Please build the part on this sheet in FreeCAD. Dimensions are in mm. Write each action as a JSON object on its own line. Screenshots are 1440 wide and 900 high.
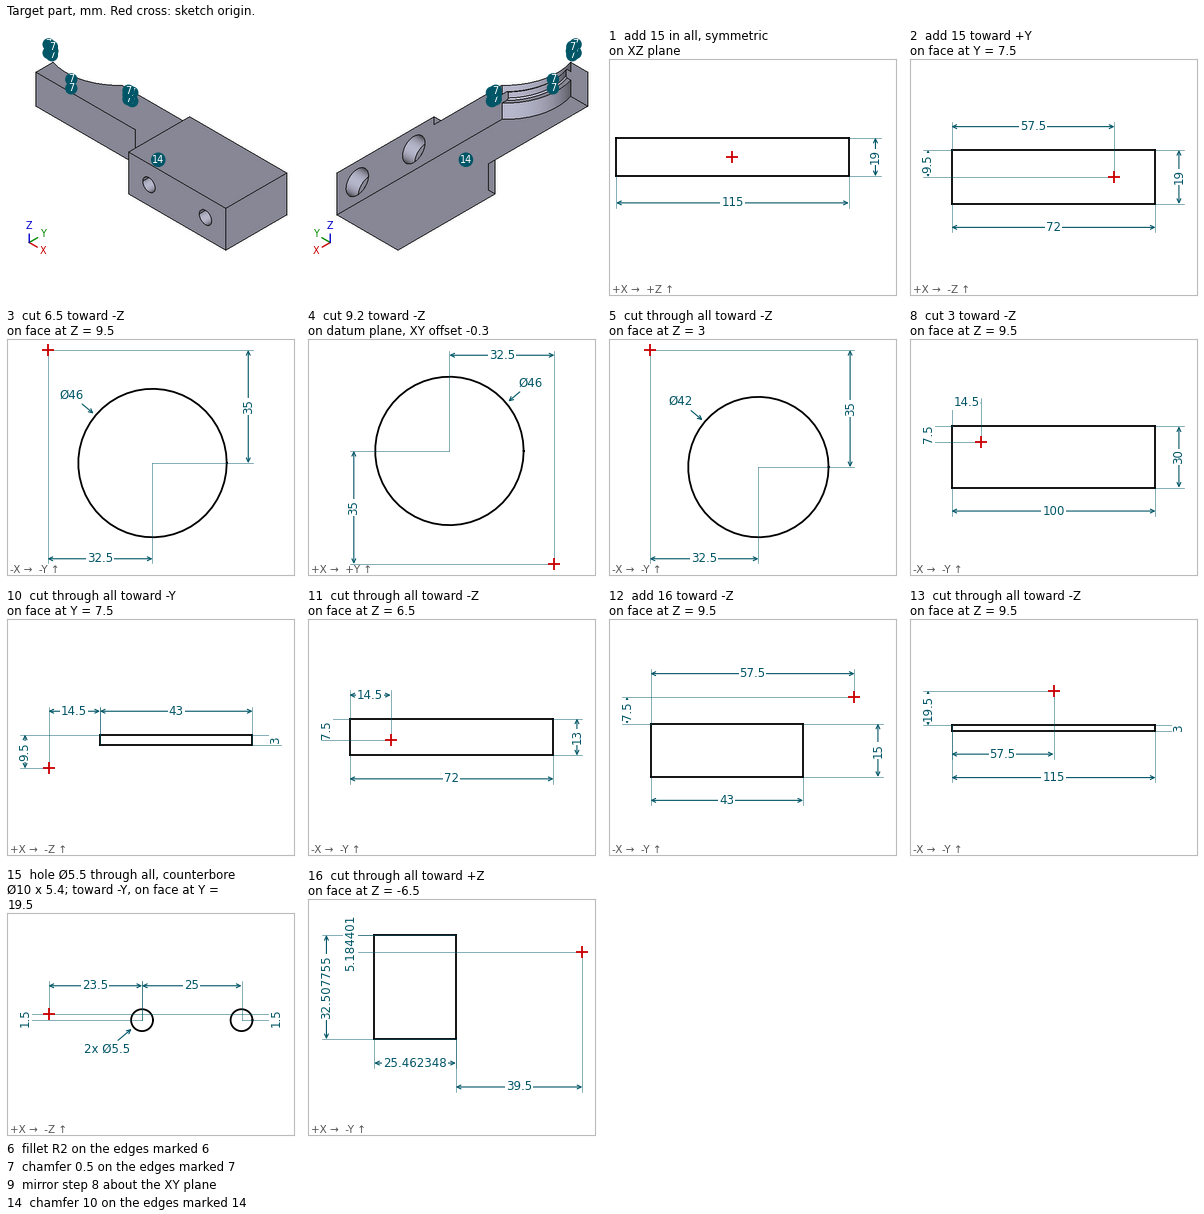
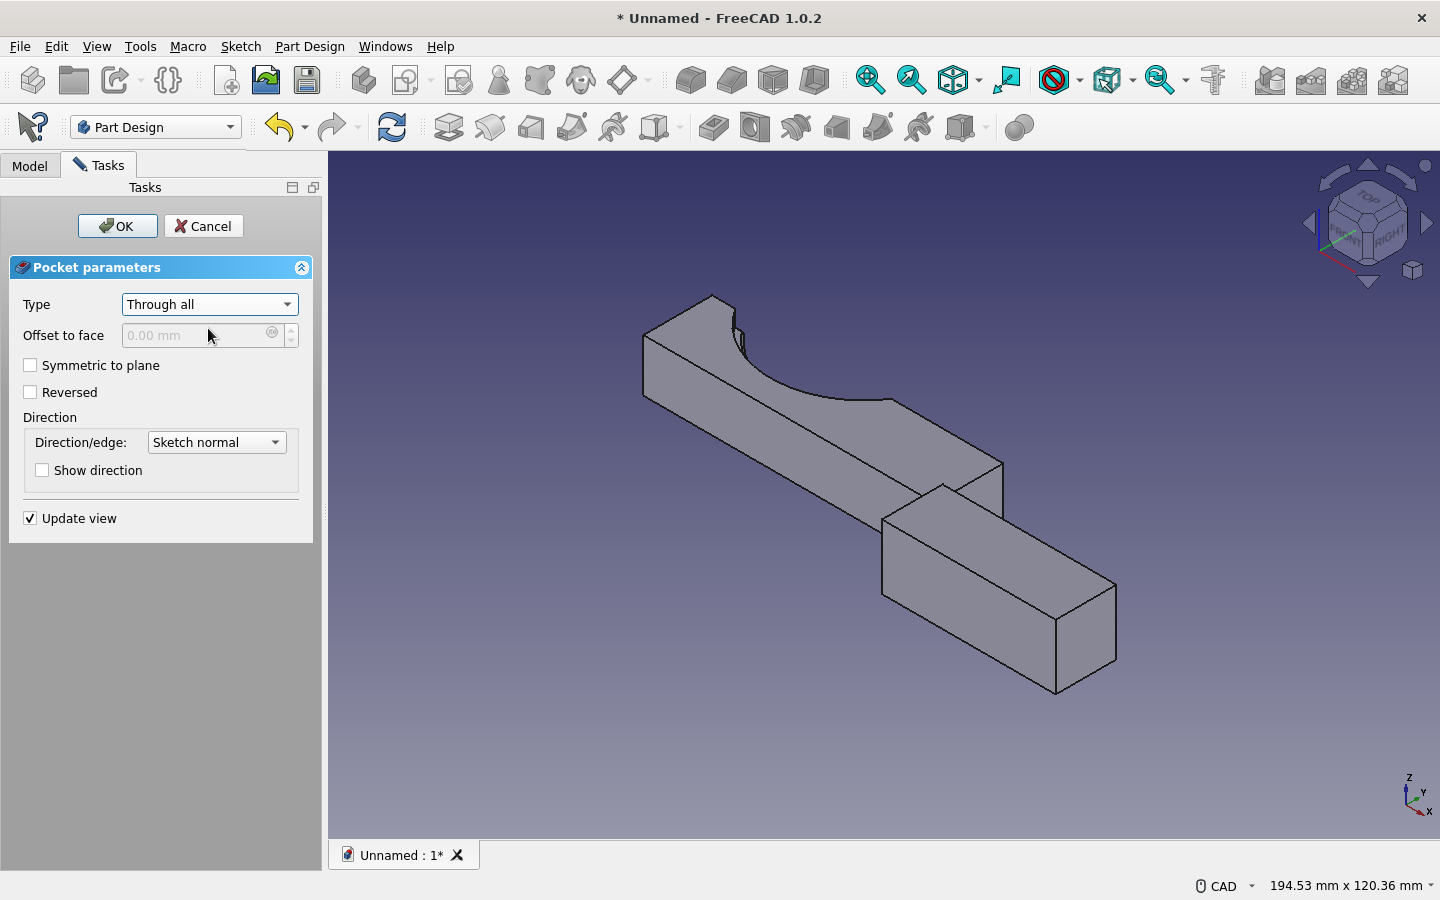
{"action": "left_click", "coordinate": [118, 226]}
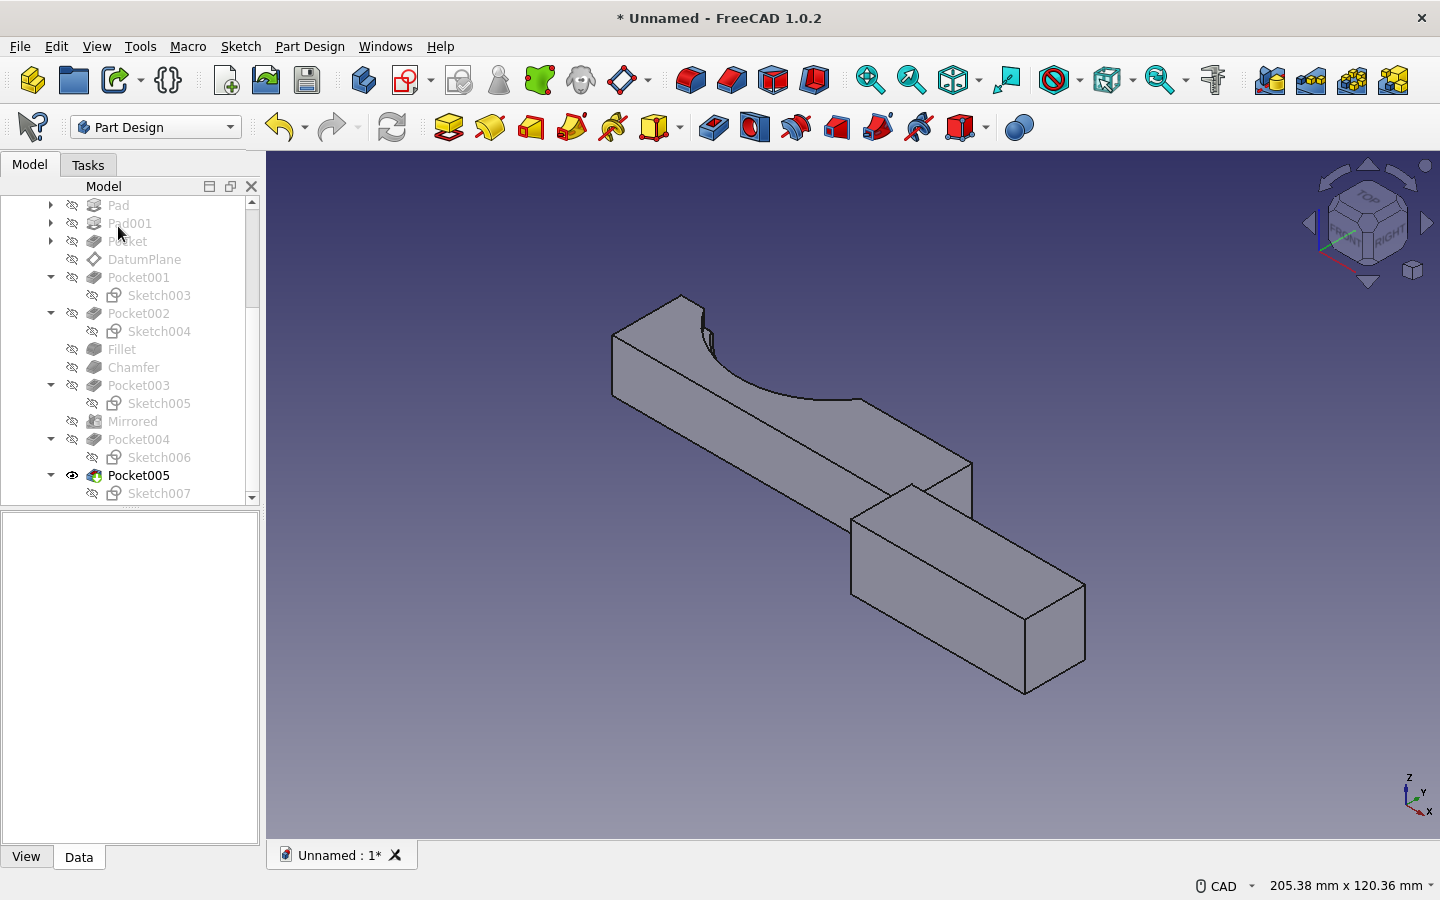
{"action": "left_click", "coordinate": [1018, 580]}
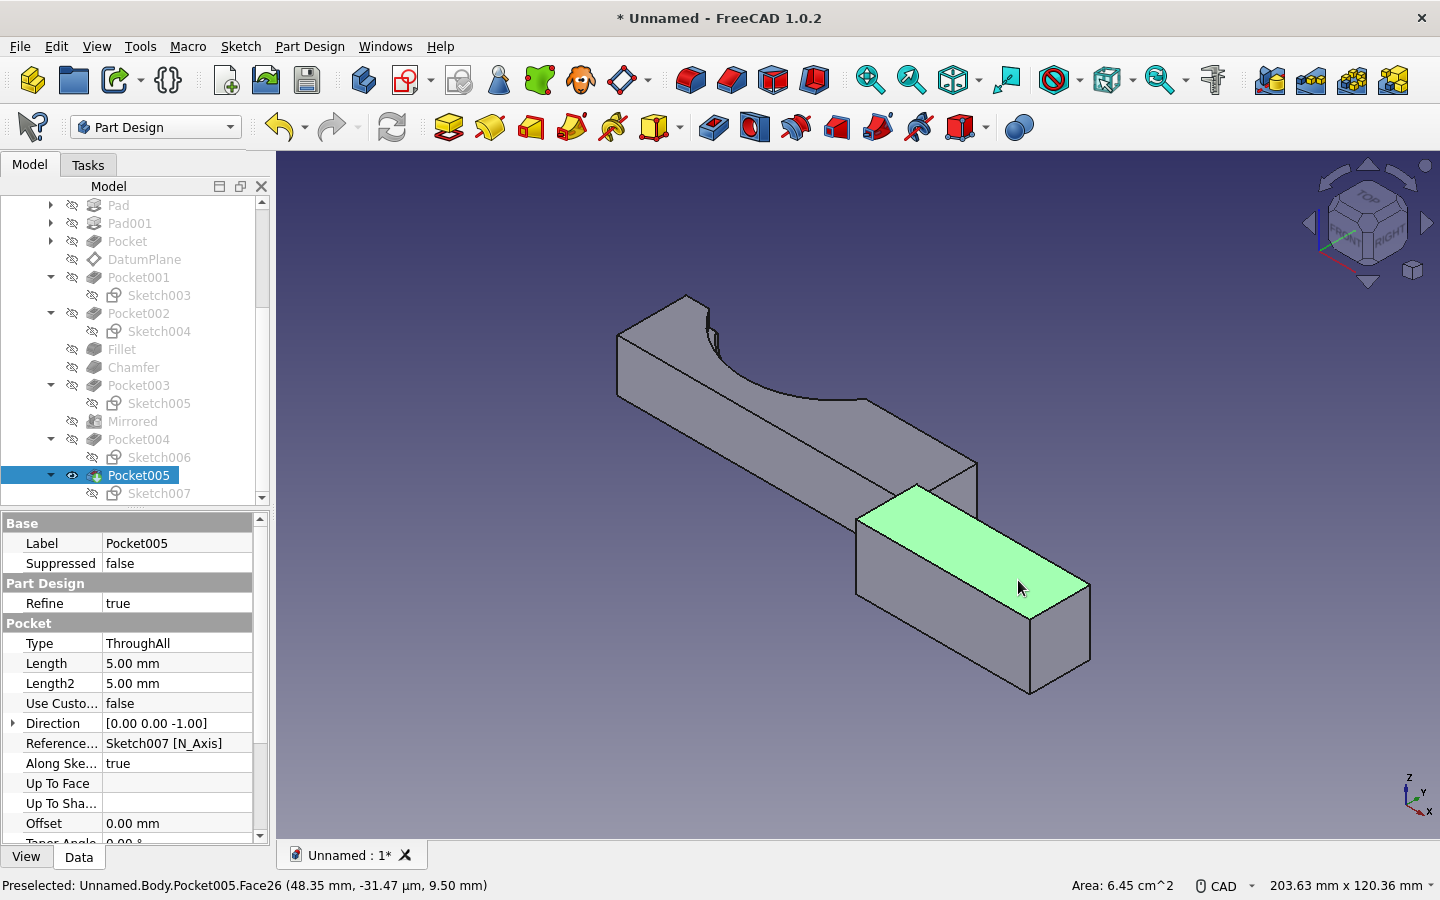
{"action": "left_click", "coordinate": [404, 80]}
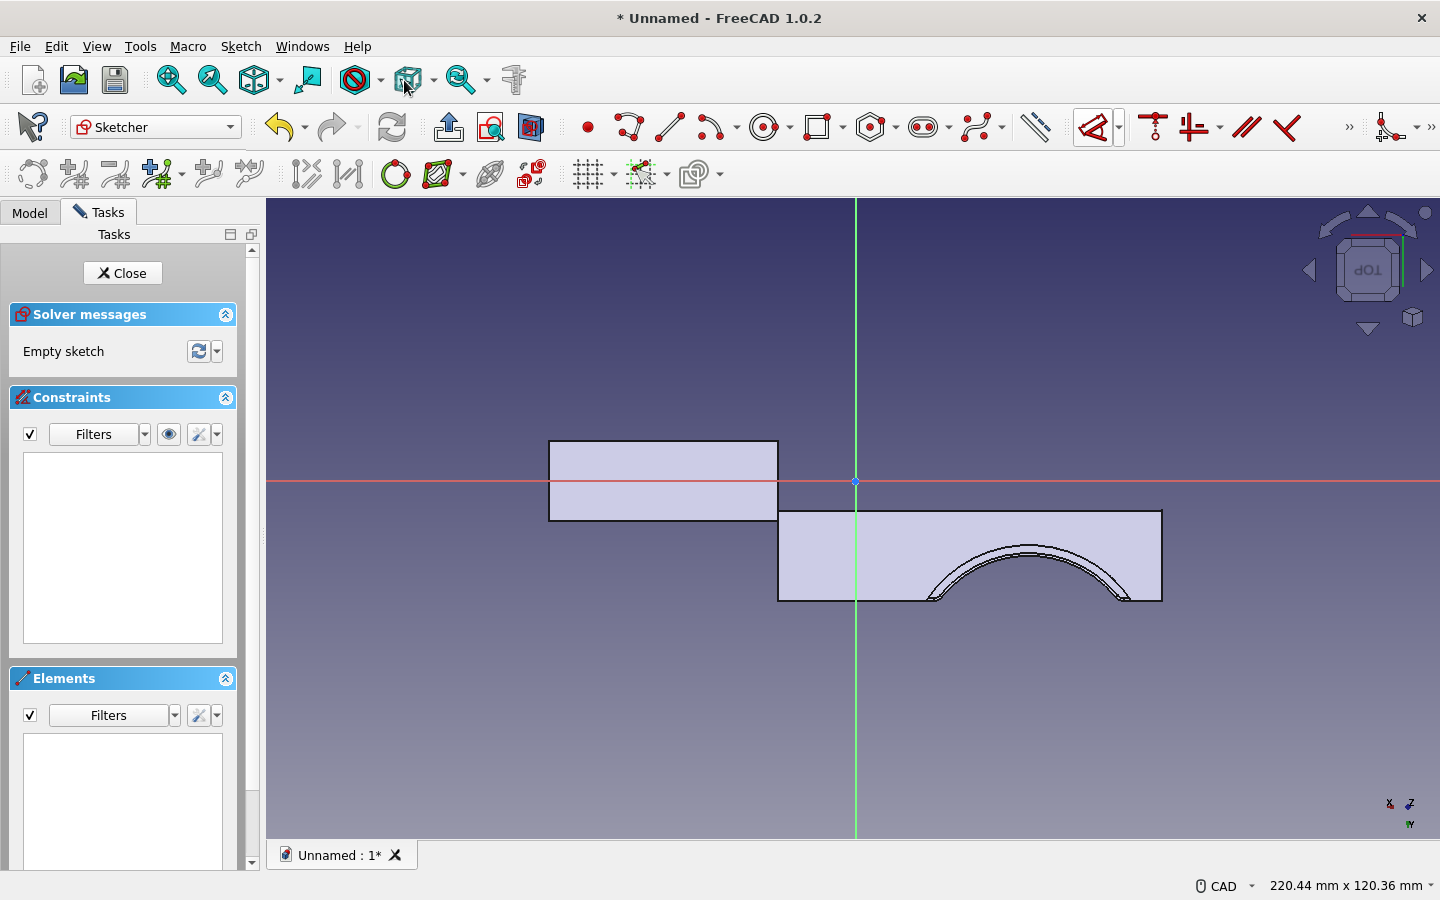
{"action": "scroll", "coordinate": [636, 560], "scroll_direction": "up", "scroll_amount": 4}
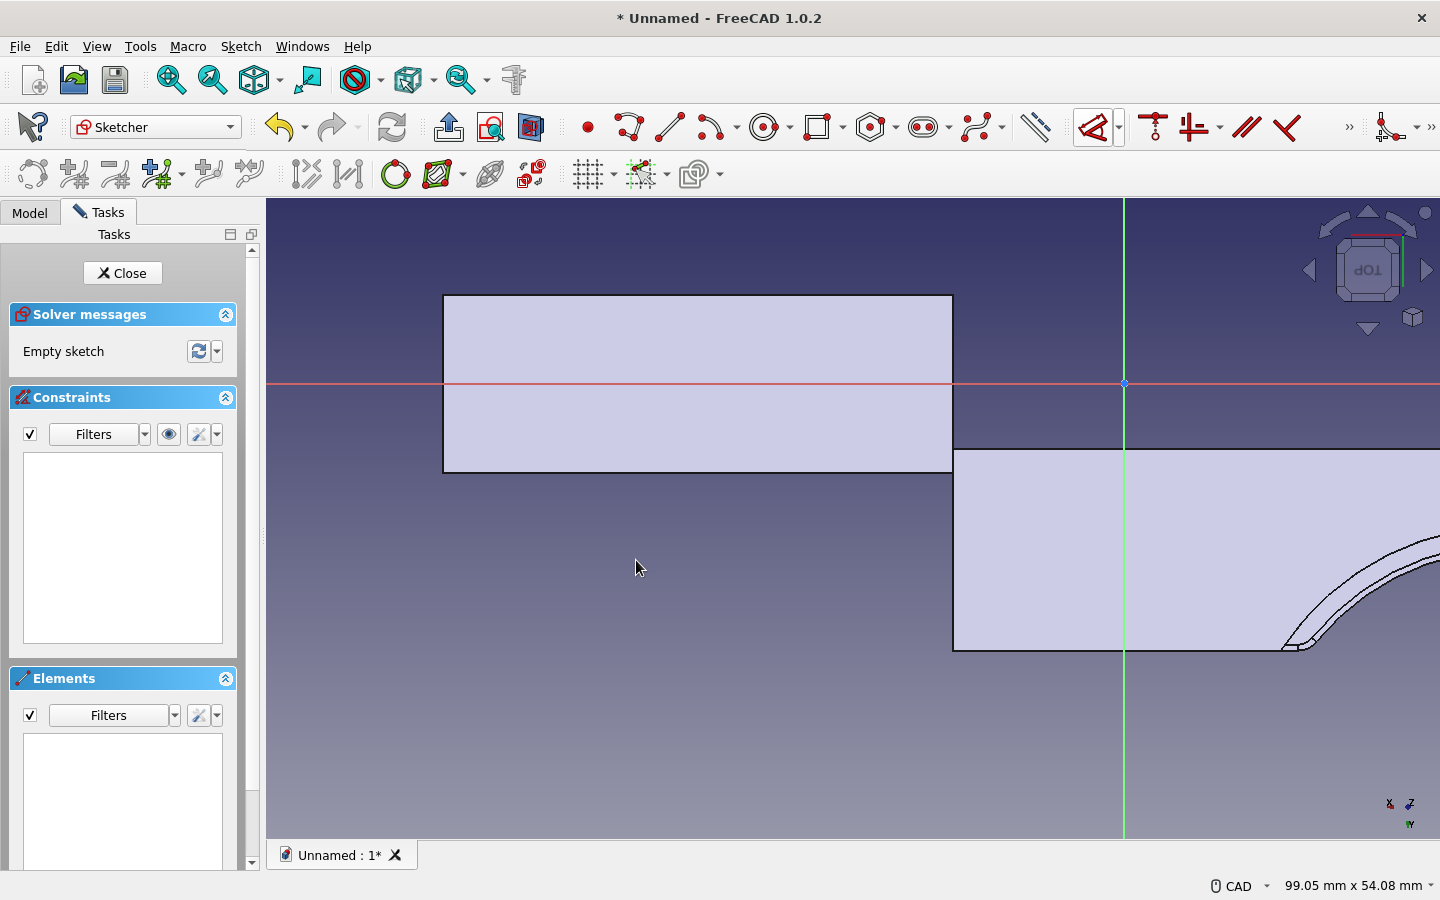
{"action": "left_click", "coordinate": [816, 128]}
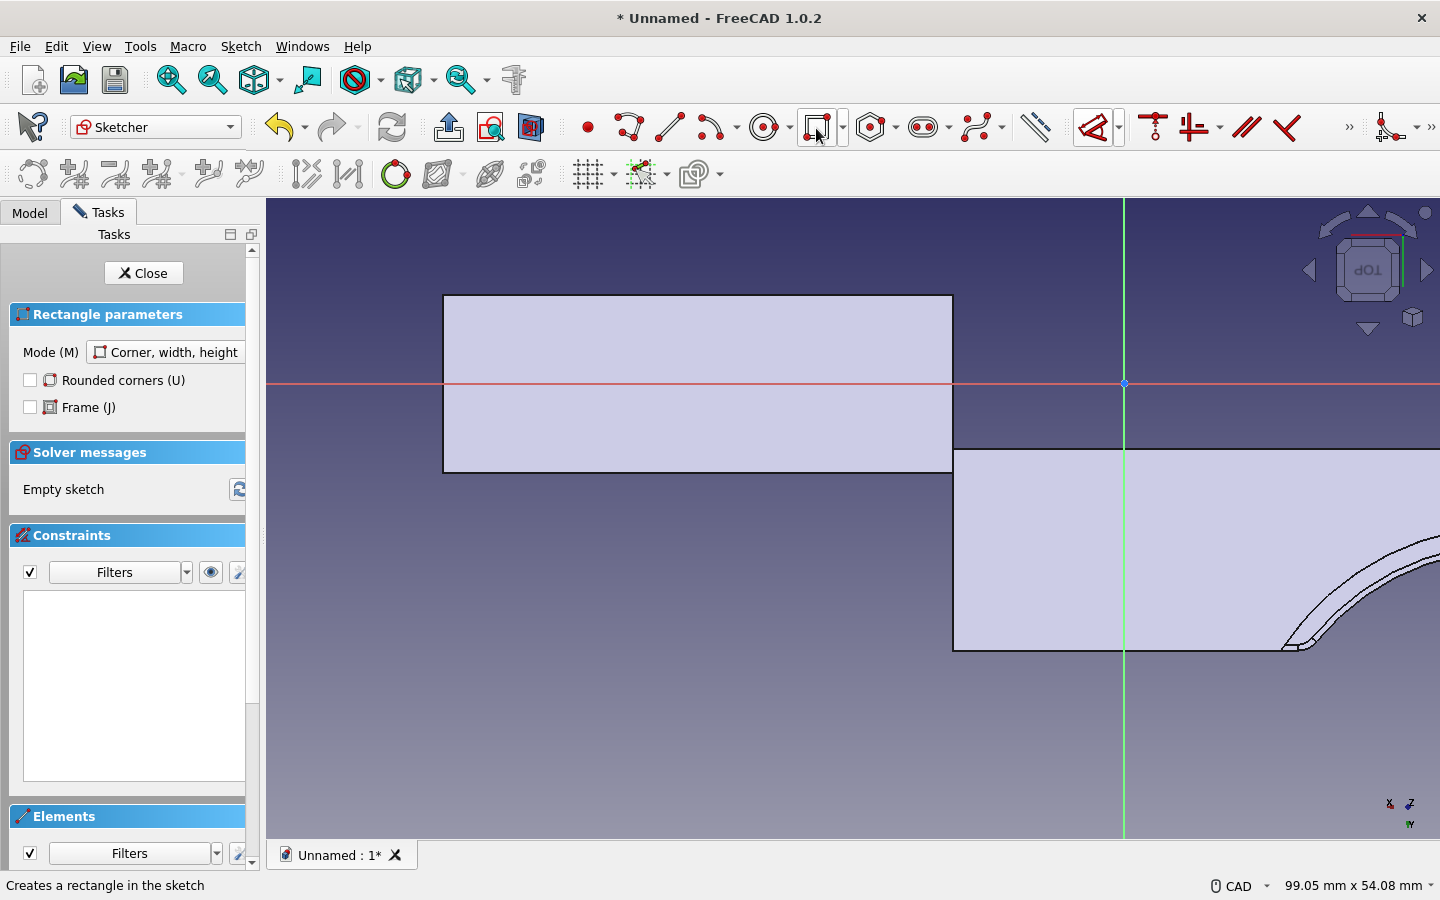
{"action": "left_click", "coordinate": [443, 473]}
{"action": "mouse_move", "coordinate": [953, 651]}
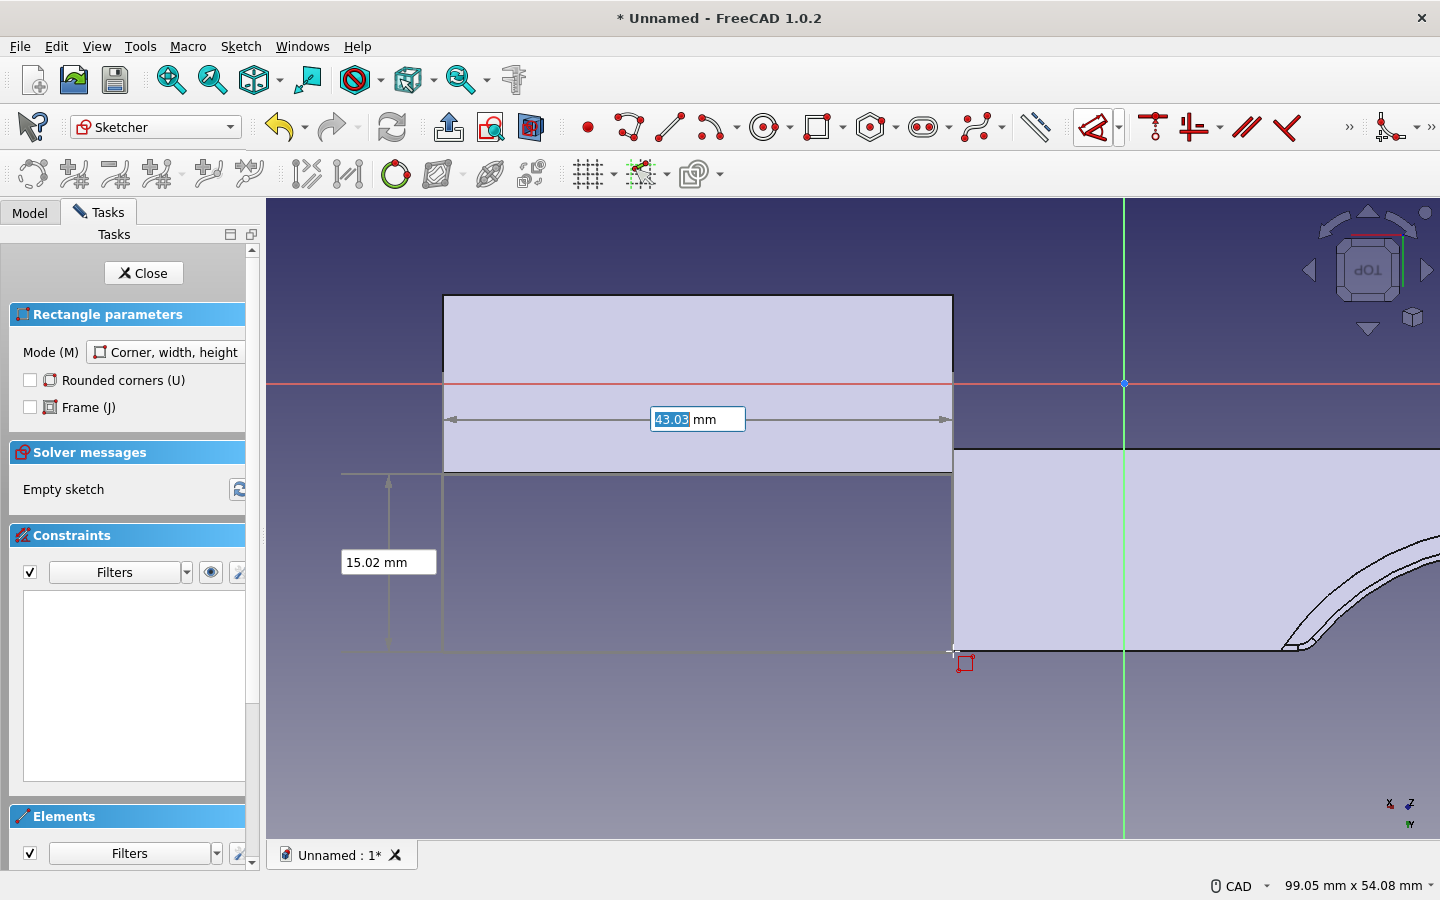
{"action": "type", "text": "43"}
{"action": "key", "text": "Tab"}
{"action": "type", "text": "15"}
{"action": "key", "text": "Return"}
{"action": "key", "text": "Escape"}